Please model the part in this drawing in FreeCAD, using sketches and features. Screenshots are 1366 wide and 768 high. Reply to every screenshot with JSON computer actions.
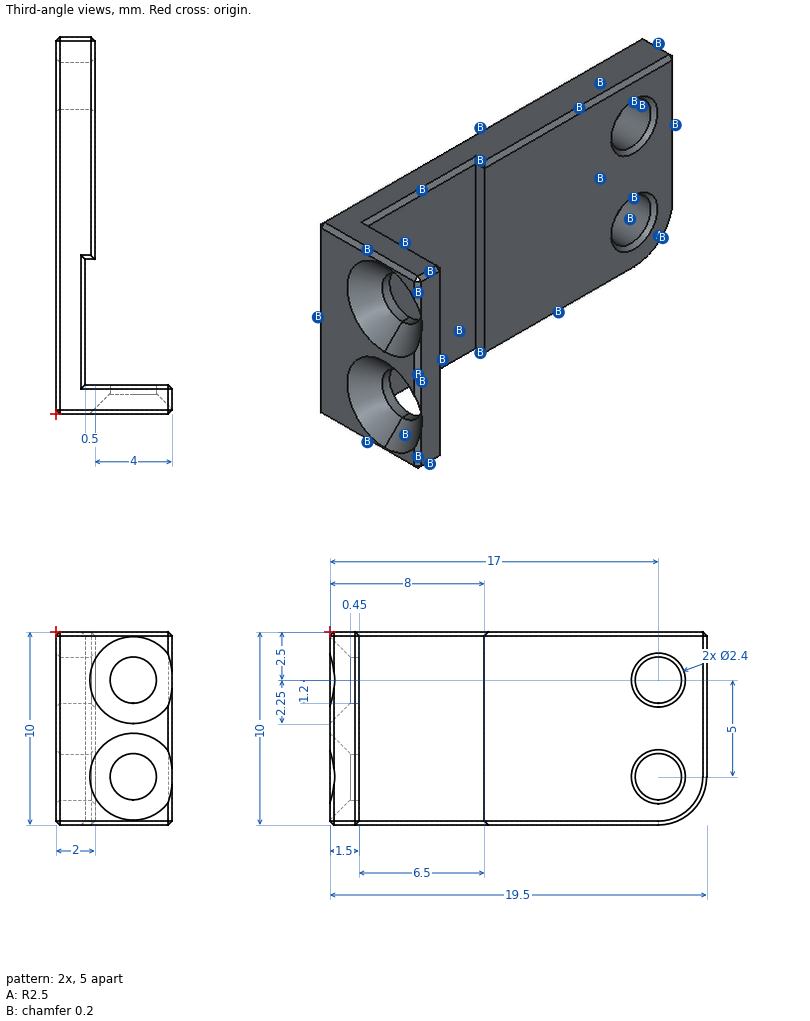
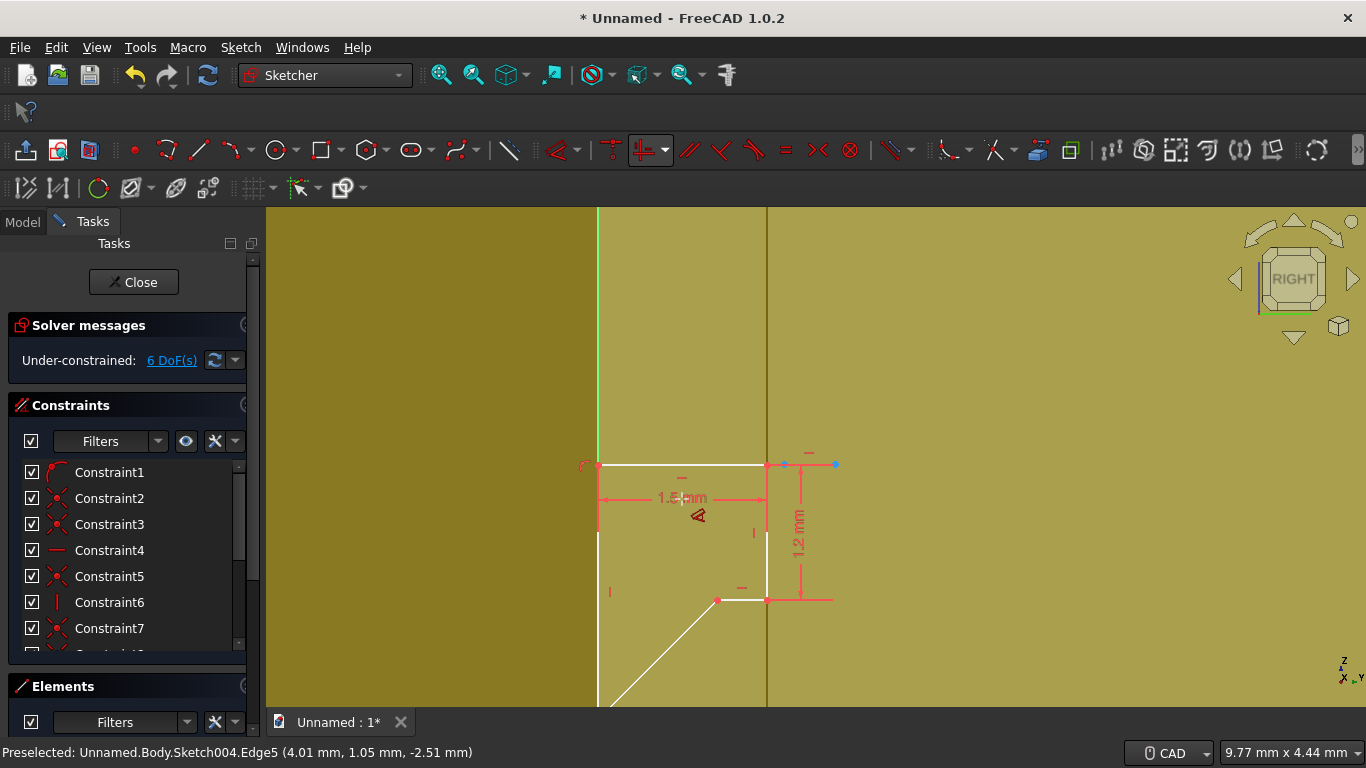
{"action": "left_click", "coordinate": [598, 541]}
{"action": "left_click", "coordinate": [564, 572]}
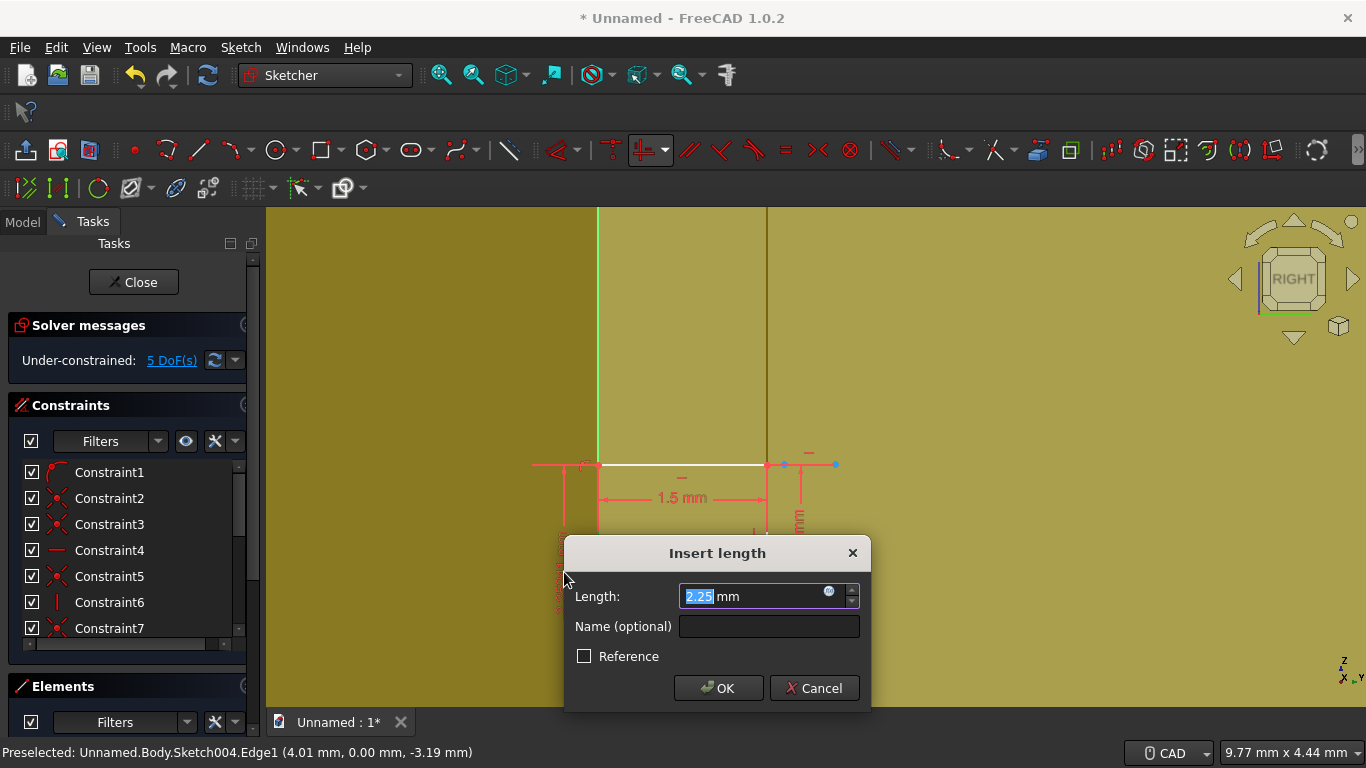
{"action": "type", "text": "2.25"}
{"action": "key", "text": "Return"}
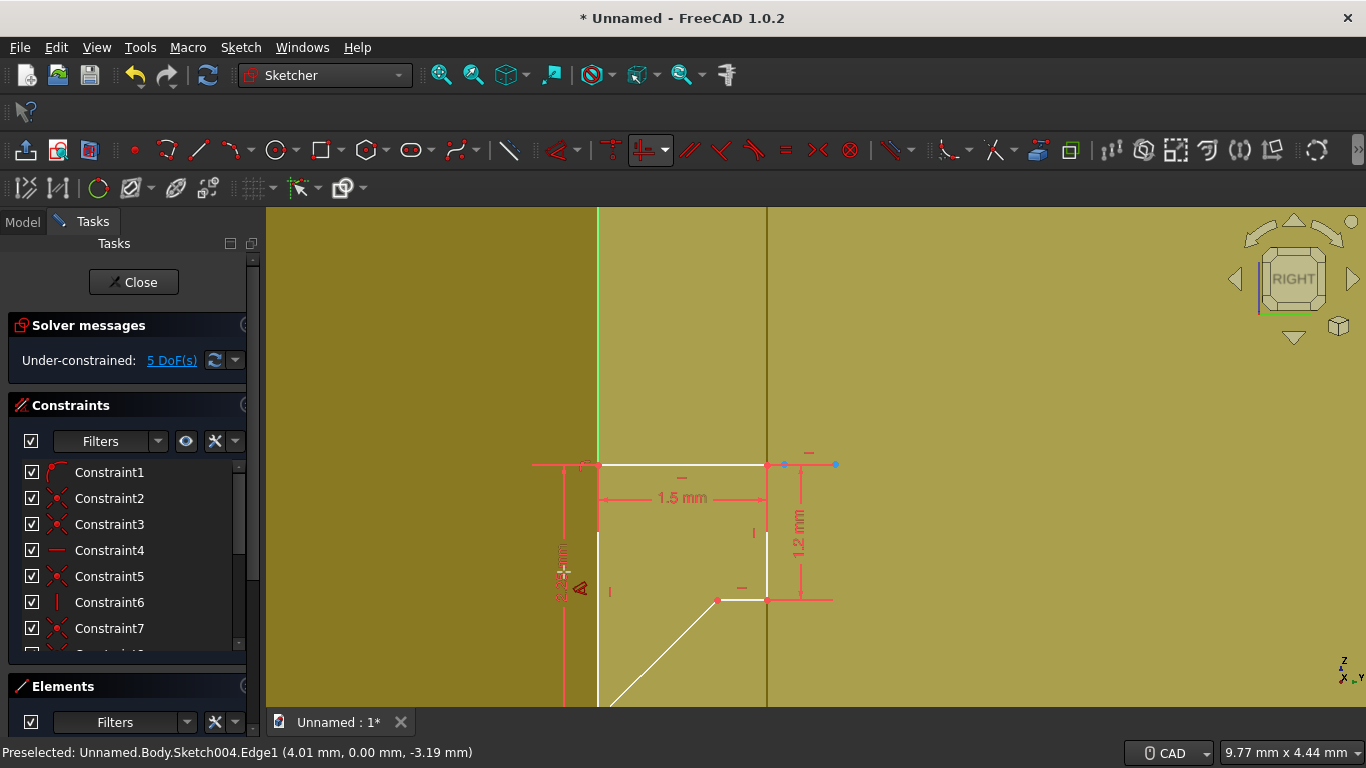
{"action": "left_click", "coordinate": [732, 600]}
{"action": "left_click", "coordinate": [742, 634]}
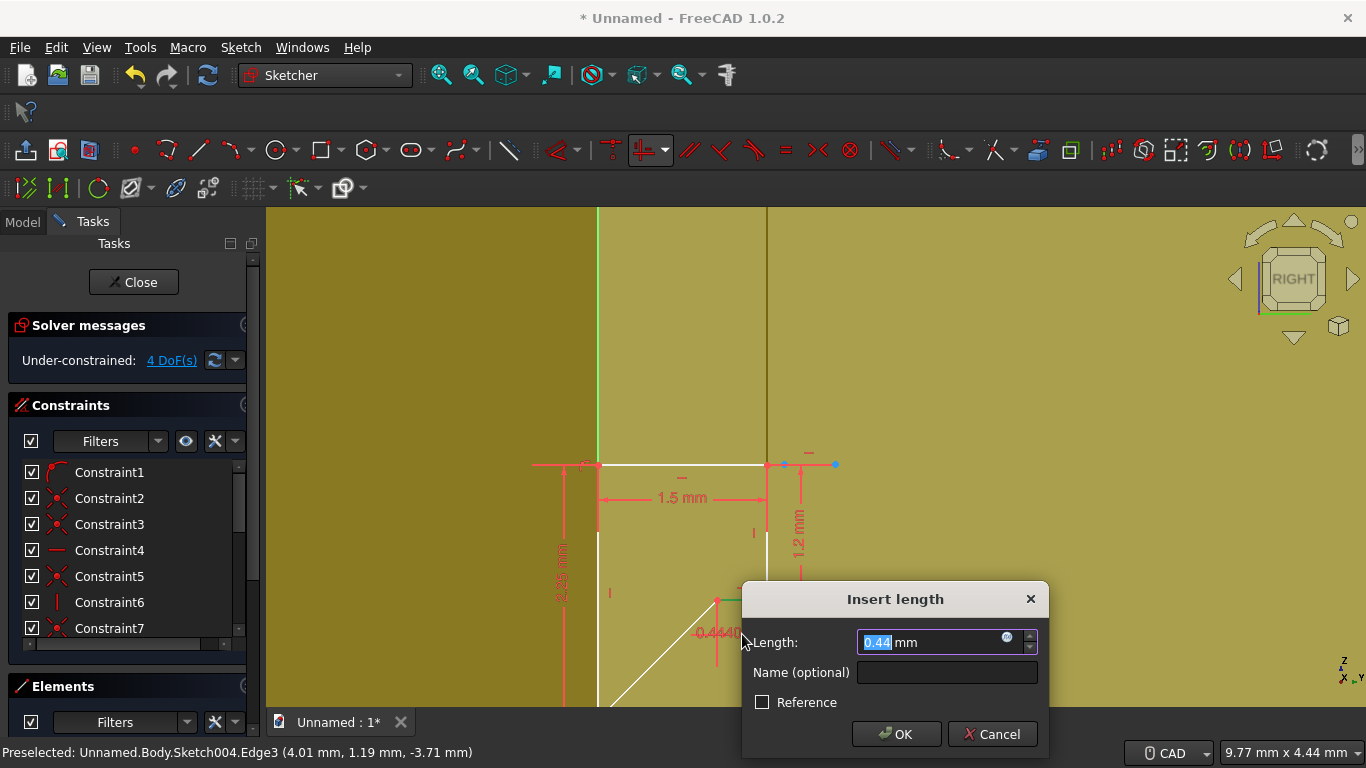
{"action": "type", "text": "0.45"}
{"action": "key", "text": "Return"}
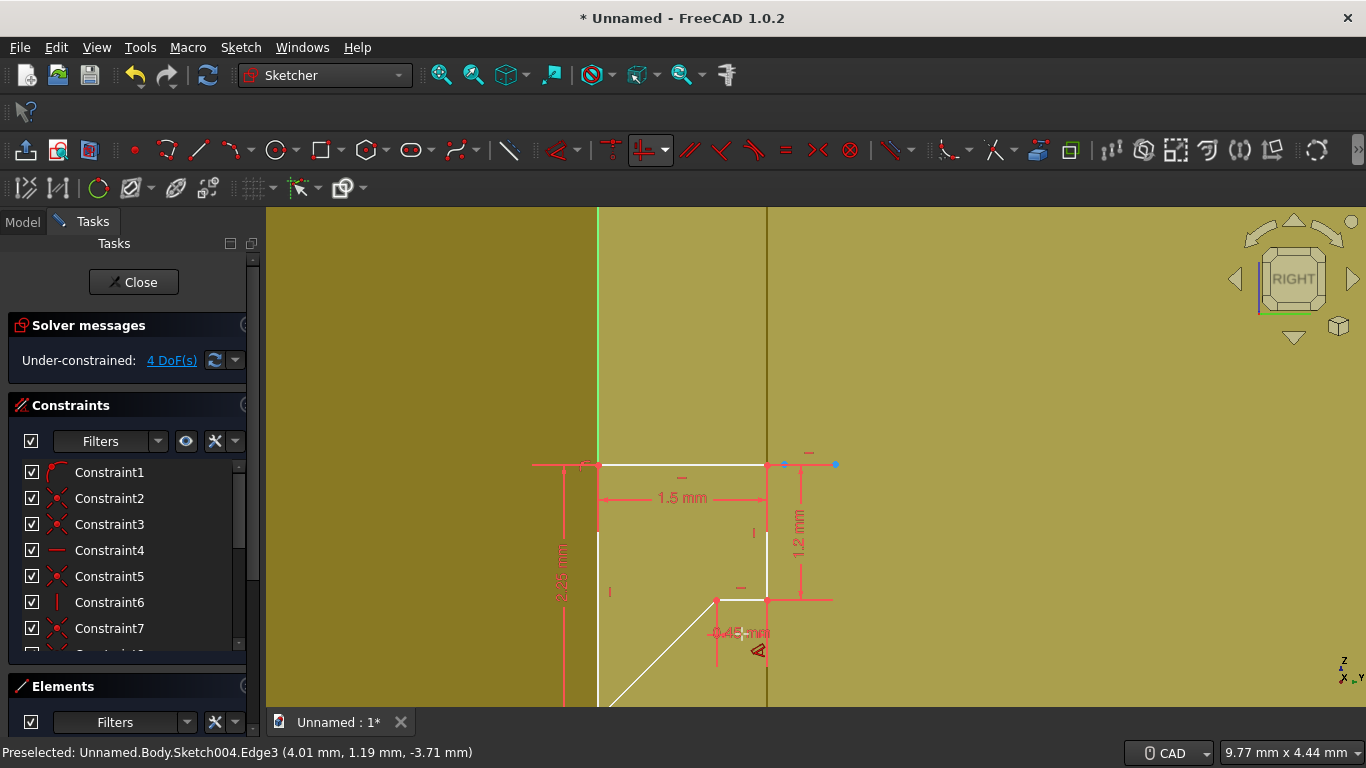
{"action": "left_click", "coordinate": [598, 465]}
{"action": "left_click", "coordinate": [564, 350]}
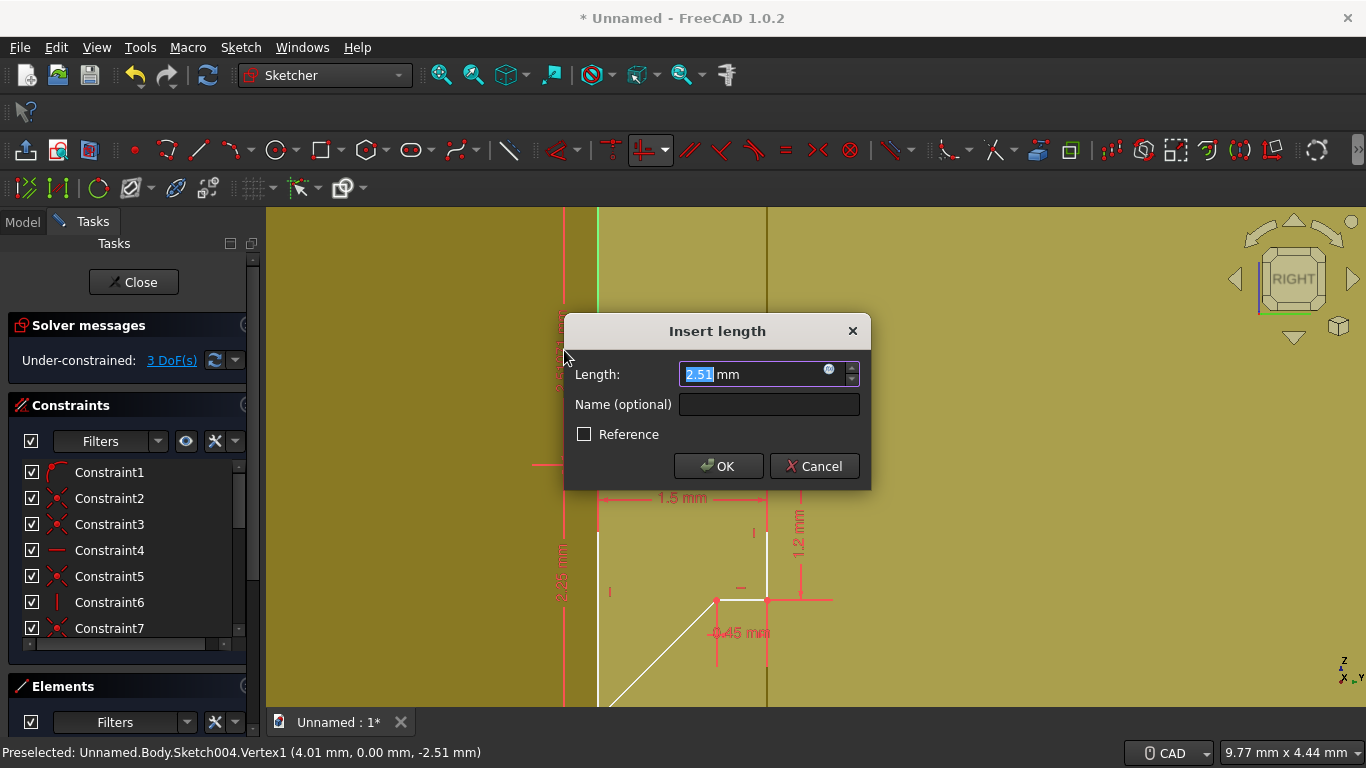
{"action": "type", "text": "2.5"}
{"action": "key", "text": "Return"}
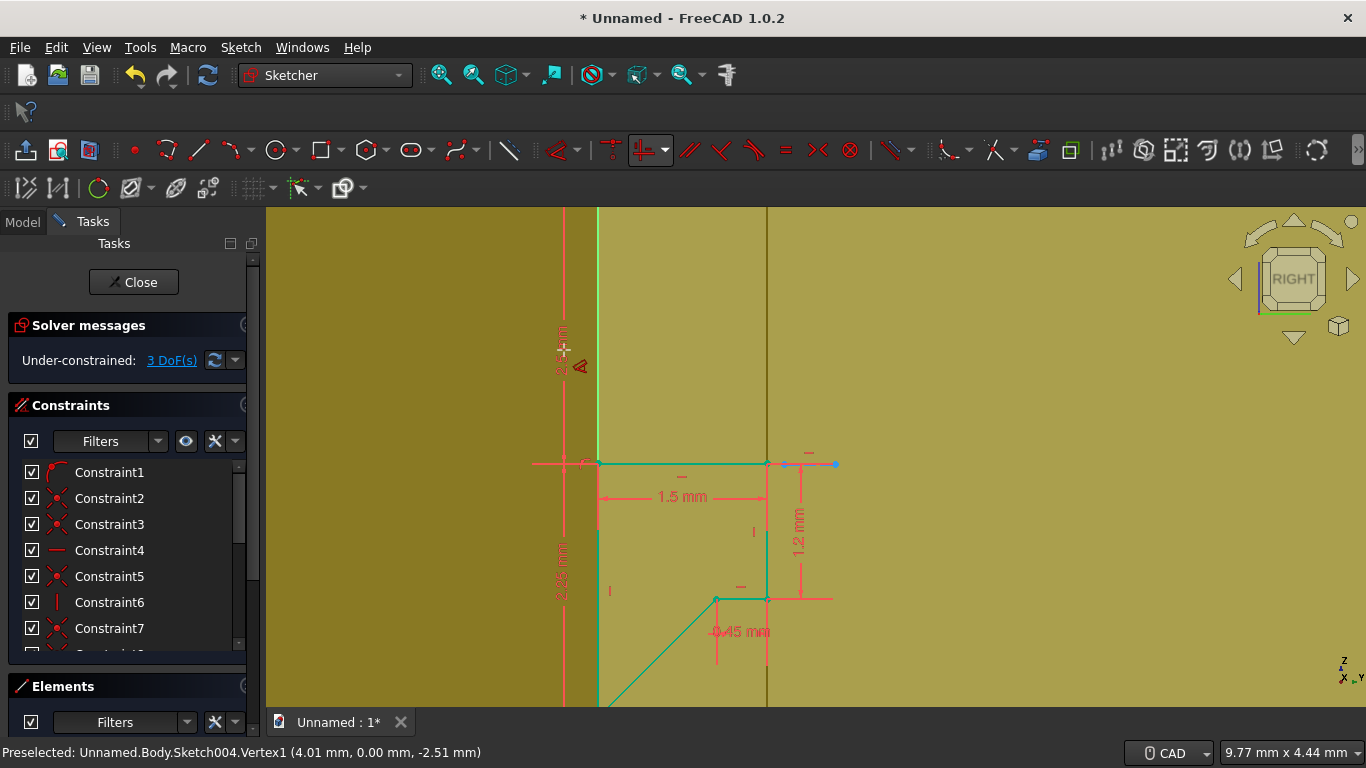
{"action": "left_click", "coordinate": [784, 465]}
{"action": "left_click", "coordinate": [564, 297]}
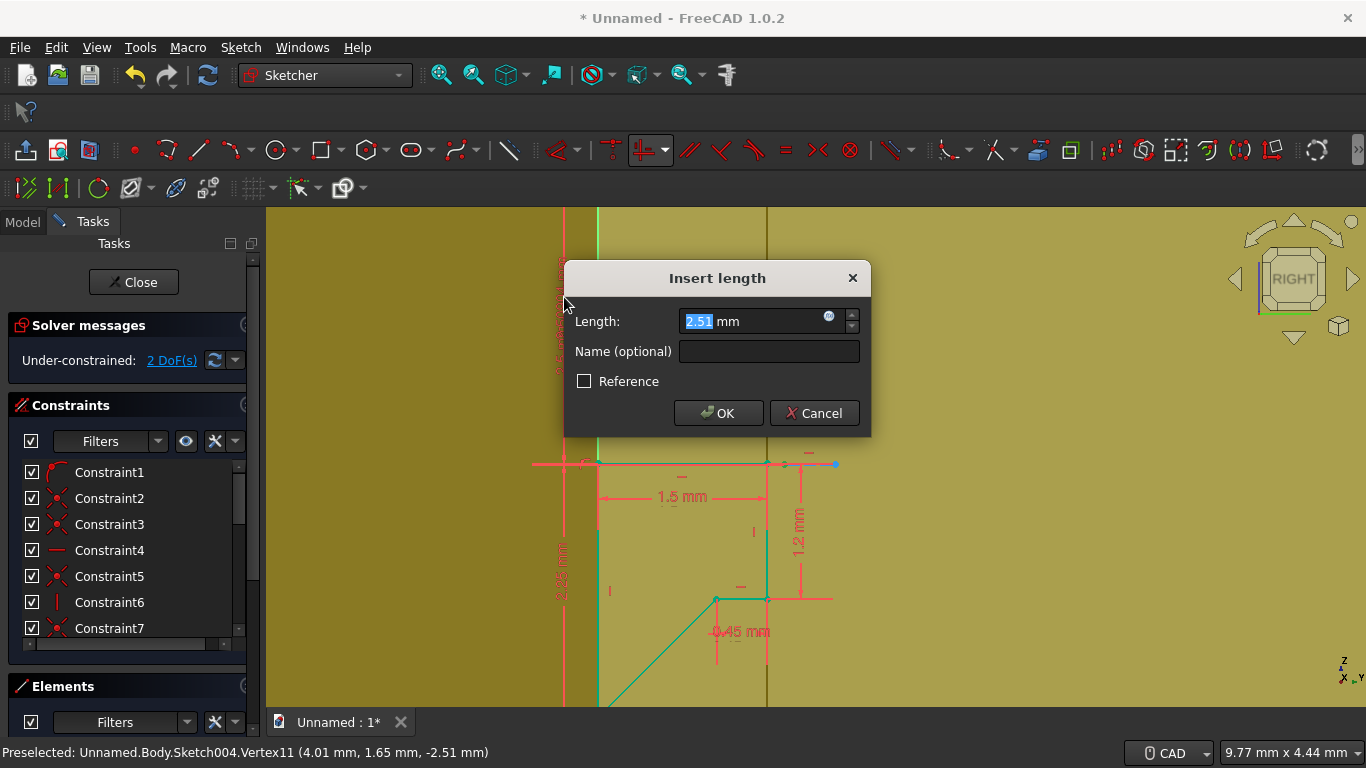
{"action": "type", "text": "2.5"}
{"action": "key", "text": "Return"}
{"action": "key", "text": "Escape"}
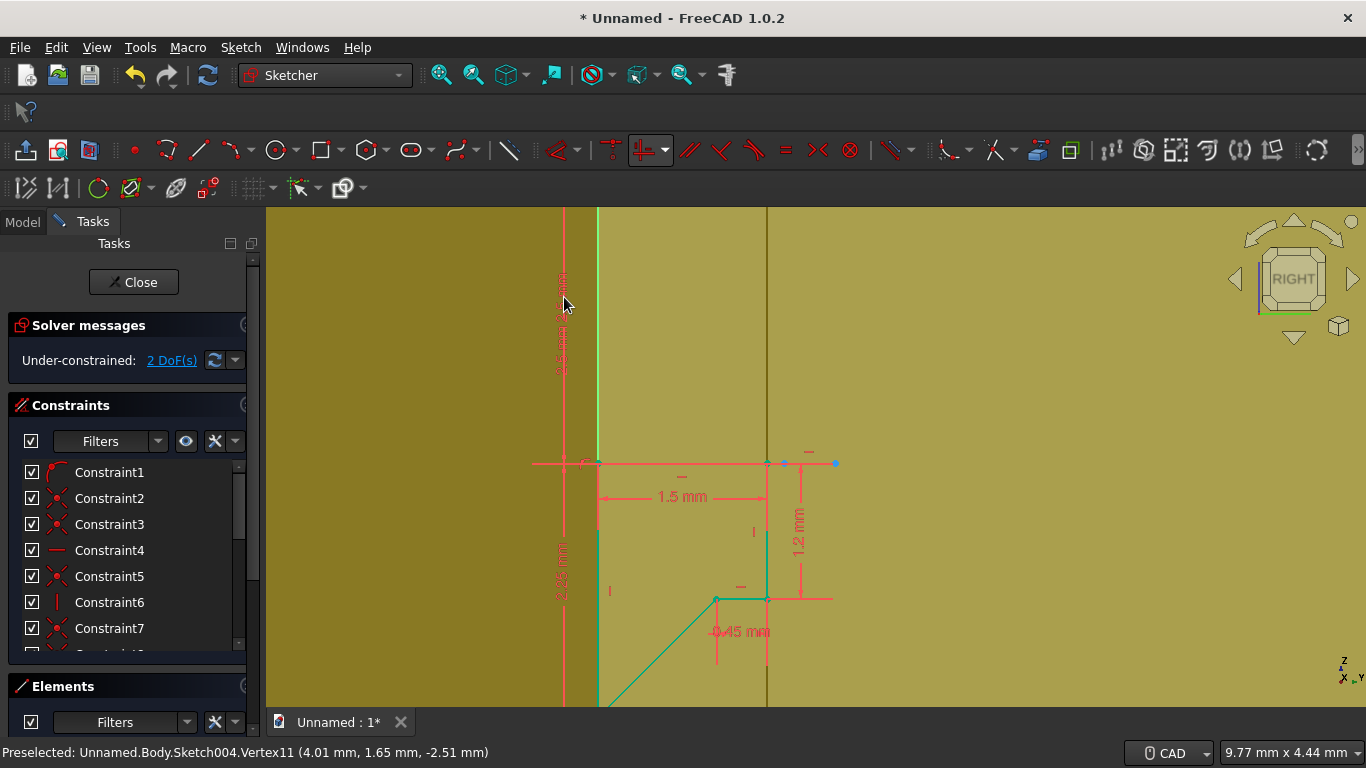
{"action": "left_click", "coordinate": [134, 282]}